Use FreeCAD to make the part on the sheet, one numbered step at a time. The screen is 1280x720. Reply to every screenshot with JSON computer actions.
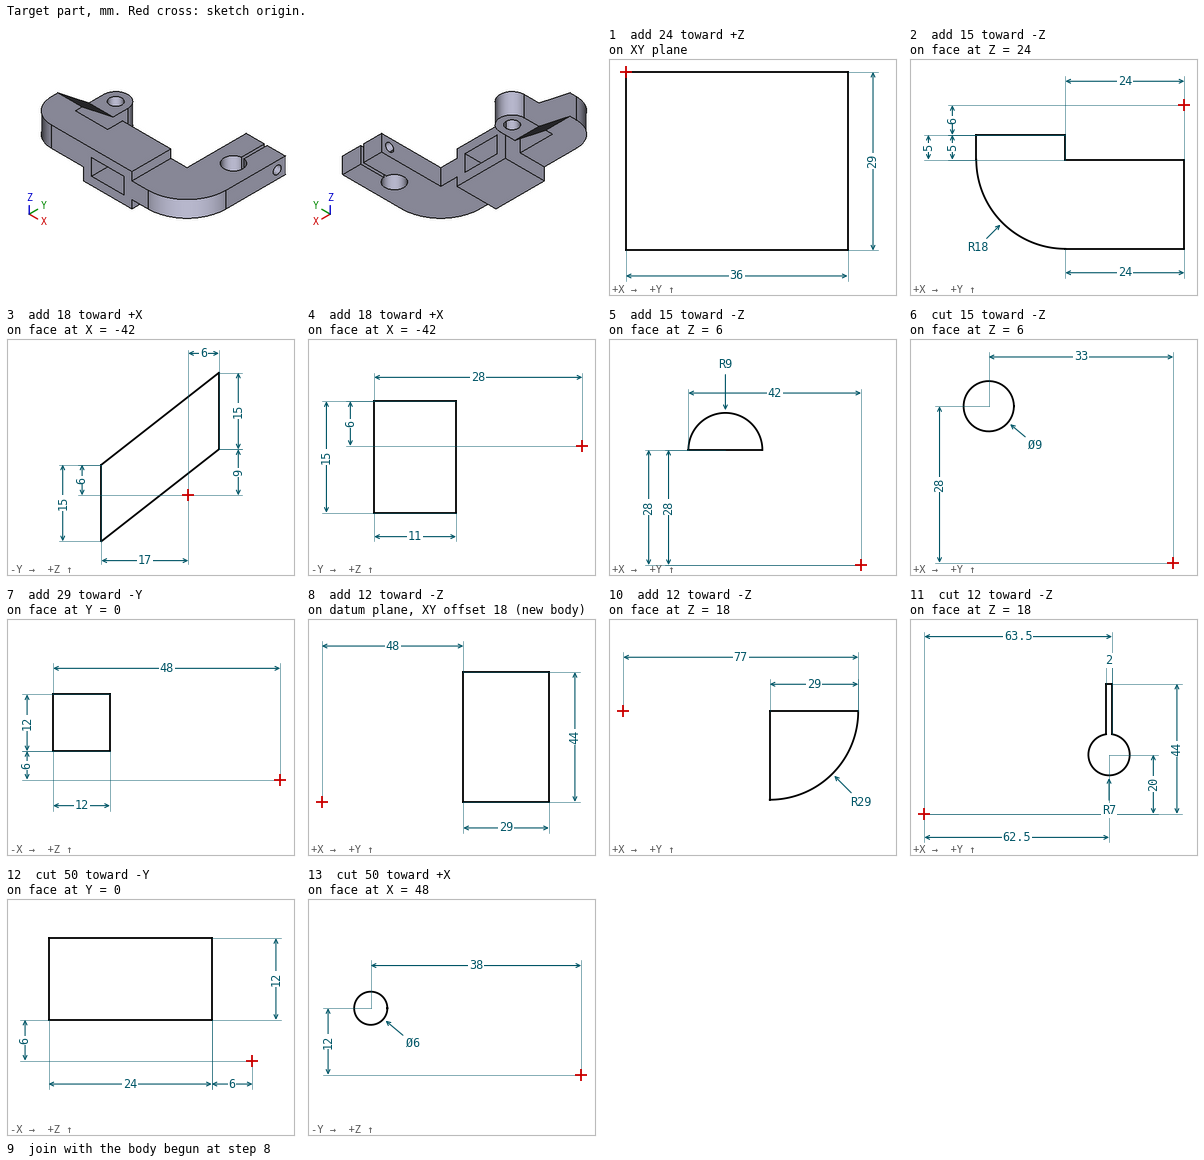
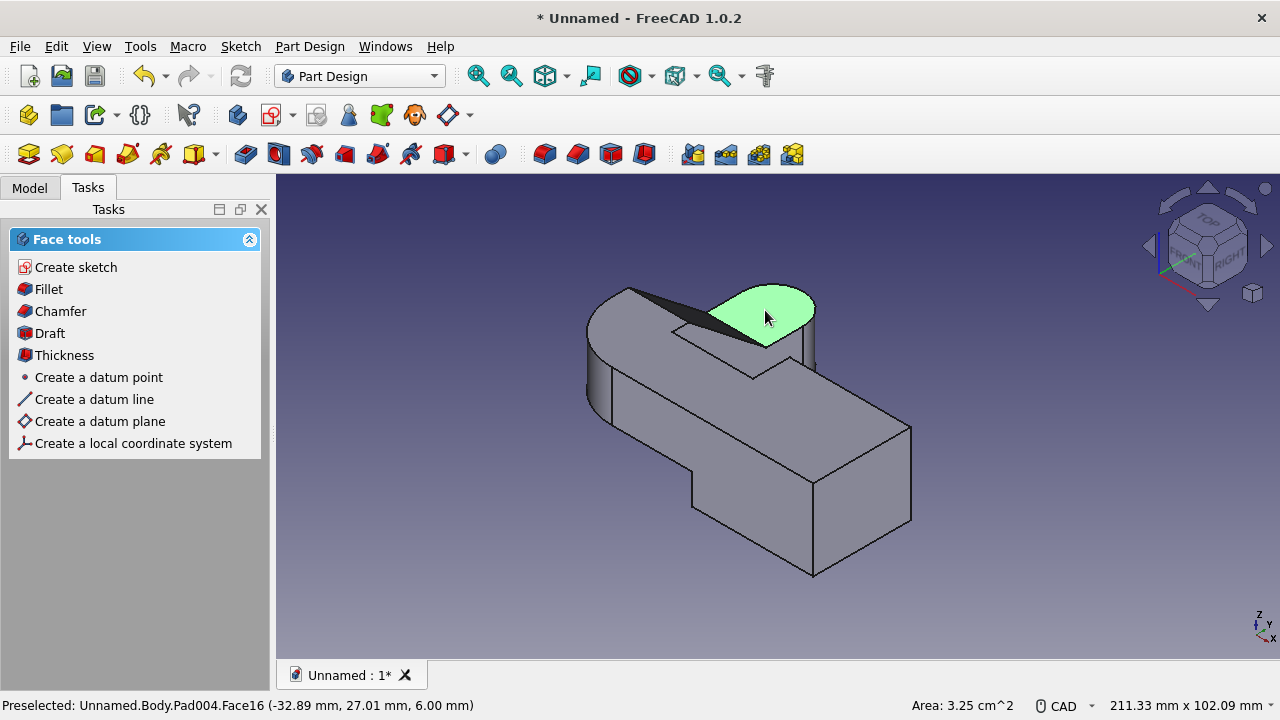
{"action": "left_click", "coordinate": [270, 116]}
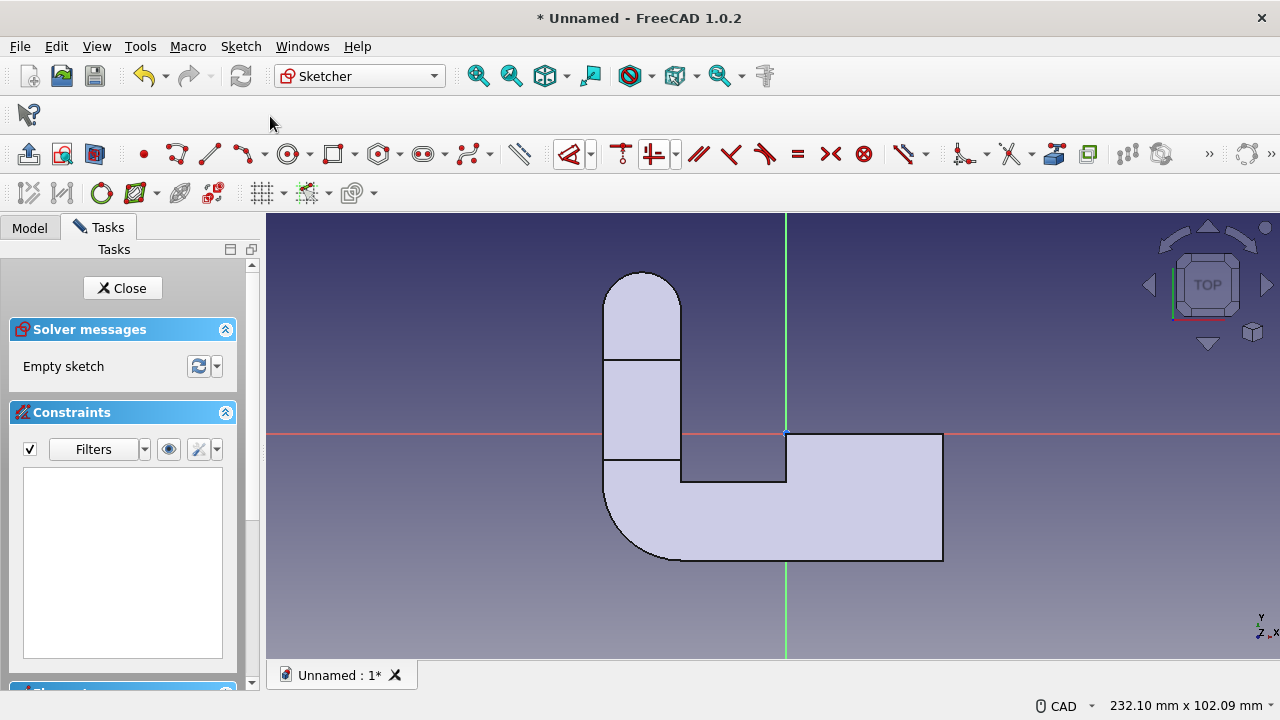
{"action": "left_click", "coordinate": [95, 154]}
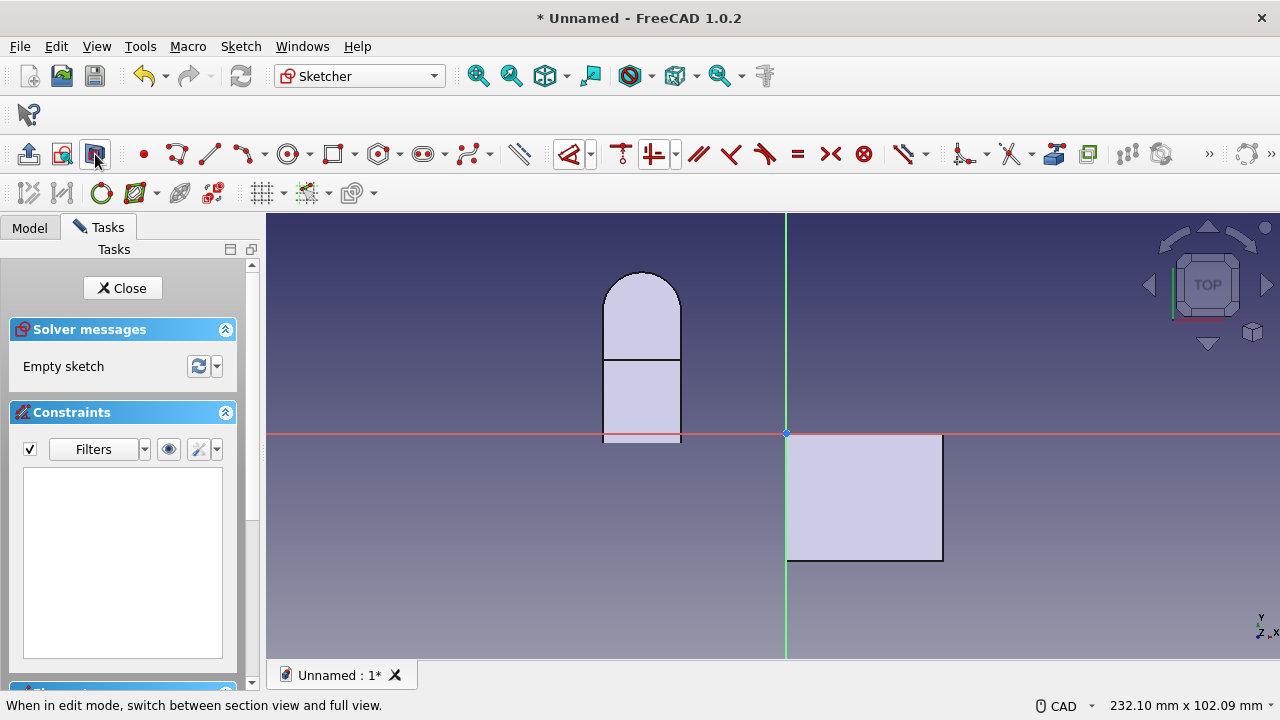
{"action": "scroll", "coordinate": [632, 292], "scroll_direction": "up", "scroll_amount": 10}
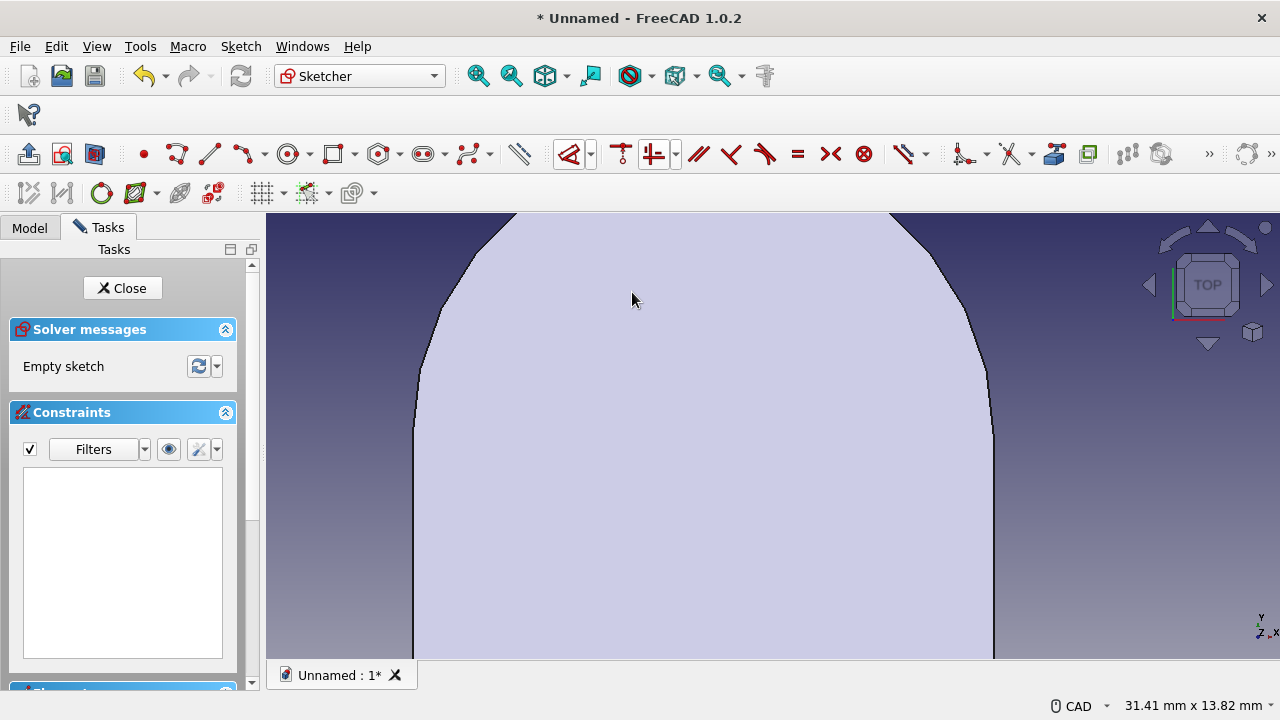
{"action": "left_click", "coordinate": [288, 154]}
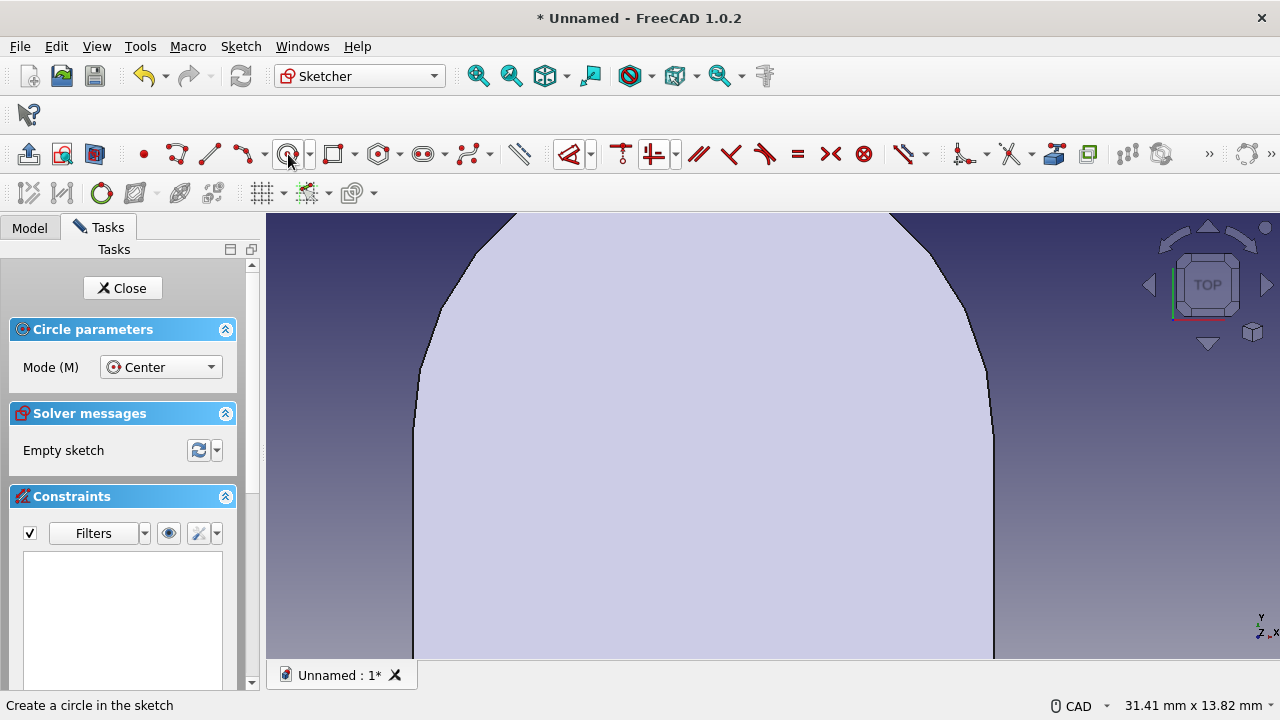
{"action": "left_click", "coordinate": [703, 435]}
{"action": "mouse_move", "coordinate": [806, 332]}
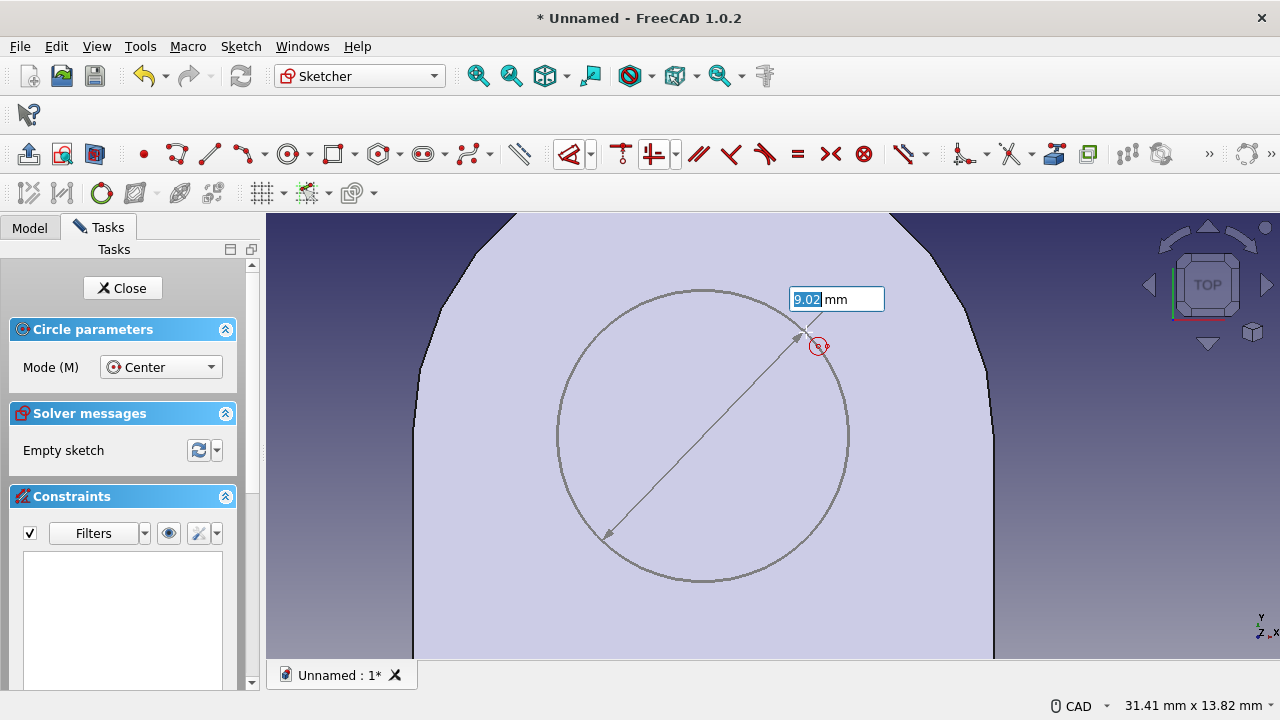
{"action": "type", "text": "9"}
{"action": "key", "text": "Return"}
{"action": "key", "text": "Escape"}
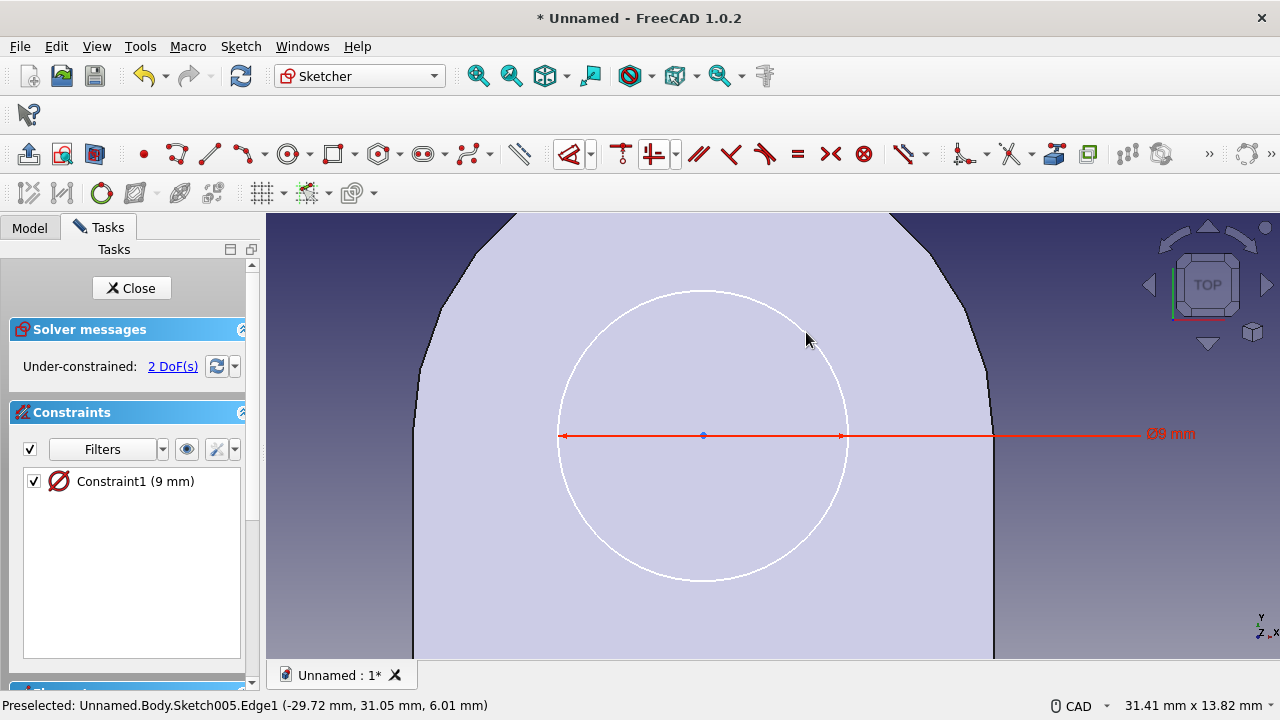
{"action": "left_click", "coordinate": [703, 436]}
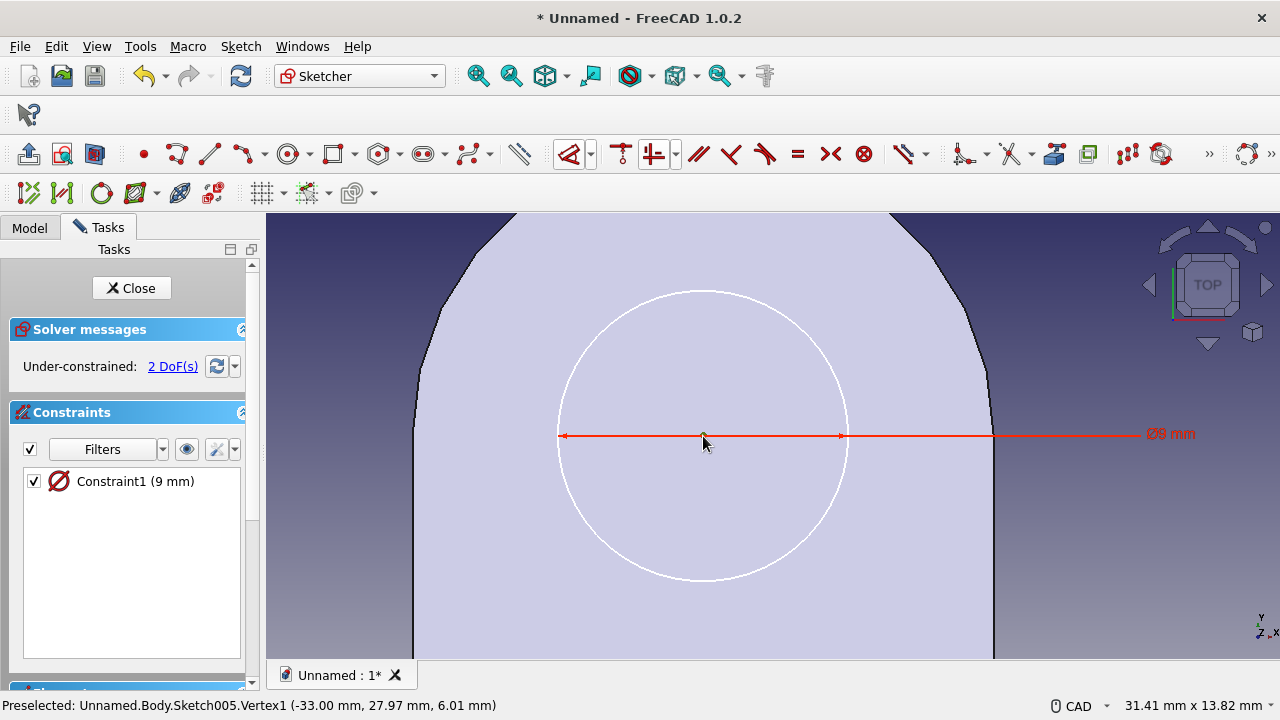
{"action": "left_click", "coordinate": [590, 154]}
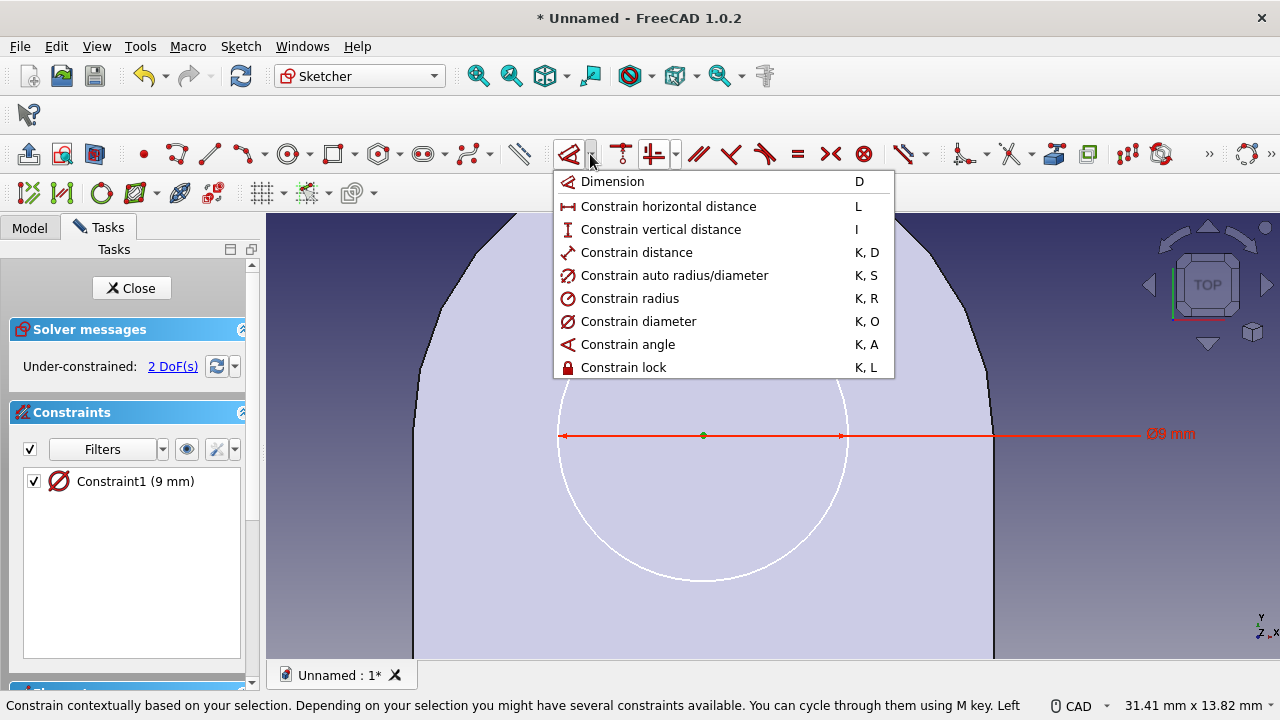
{"action": "left_click", "coordinate": [724, 206]}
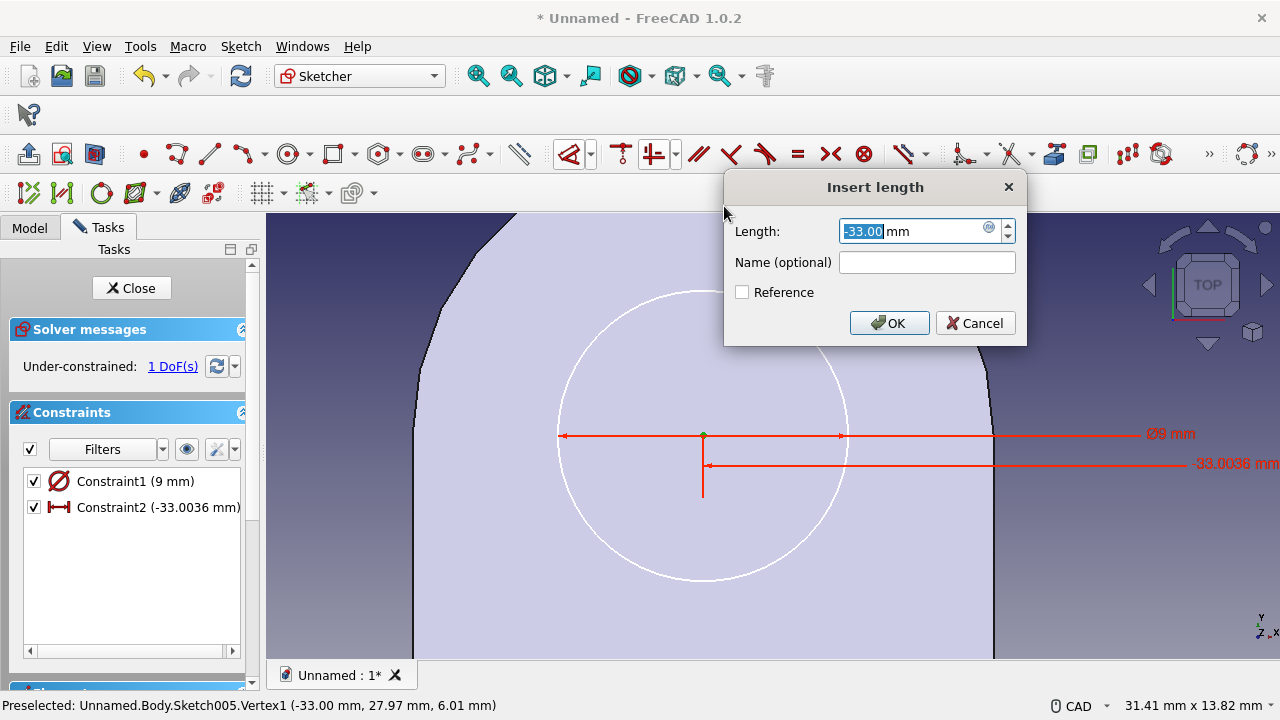
{"action": "type", "text": "-33"}
{"action": "key", "text": "Return"}